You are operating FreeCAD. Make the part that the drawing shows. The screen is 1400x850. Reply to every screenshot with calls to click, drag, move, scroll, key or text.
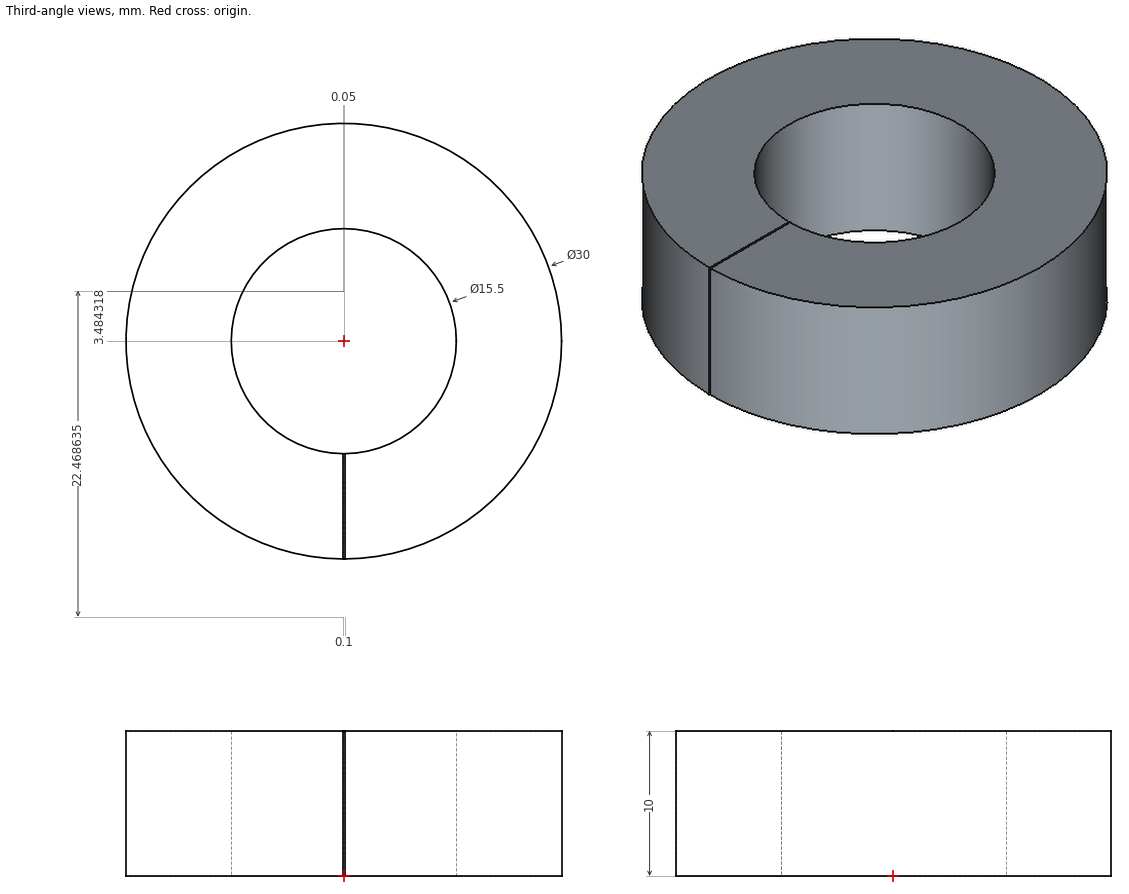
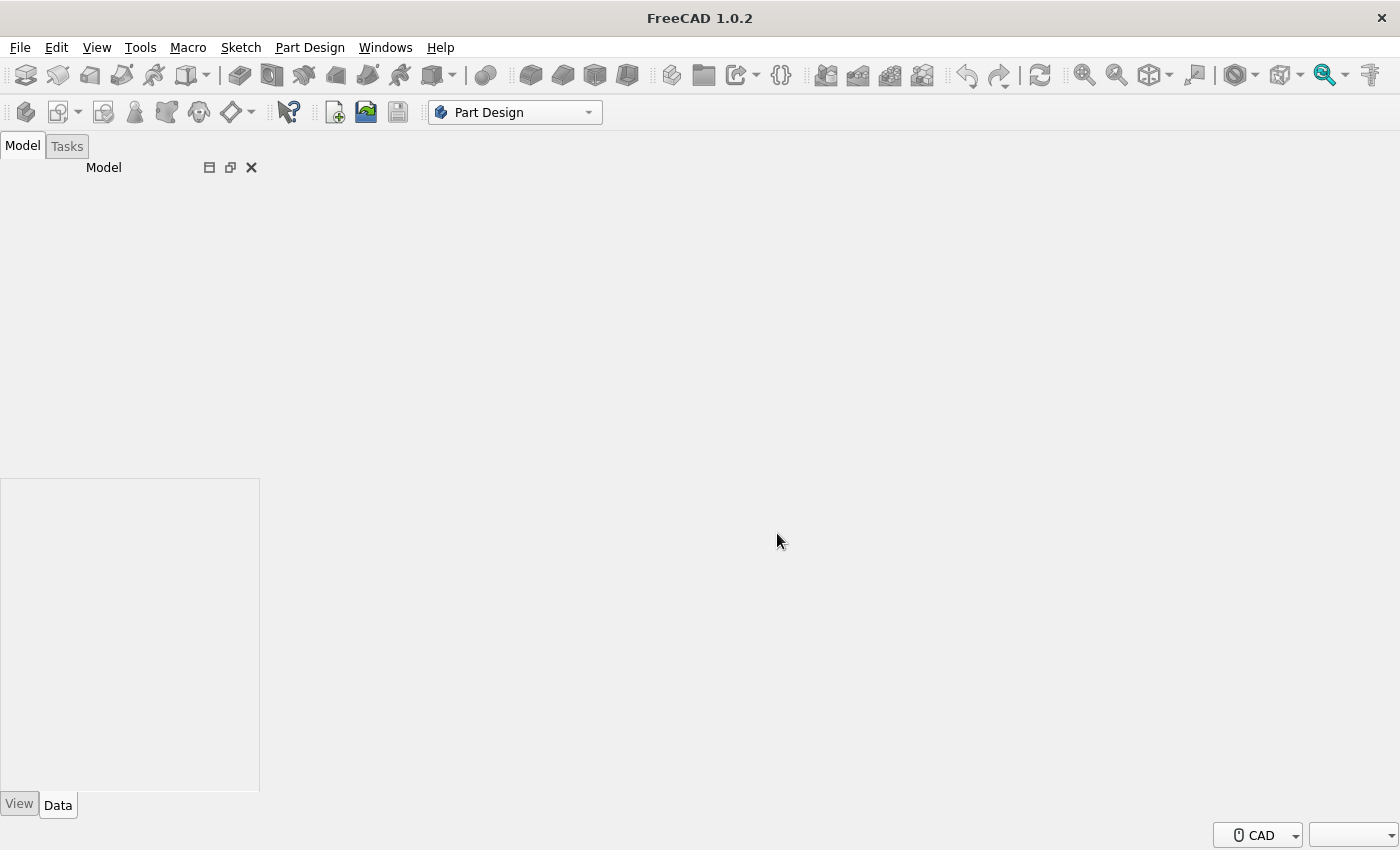
click(334, 112)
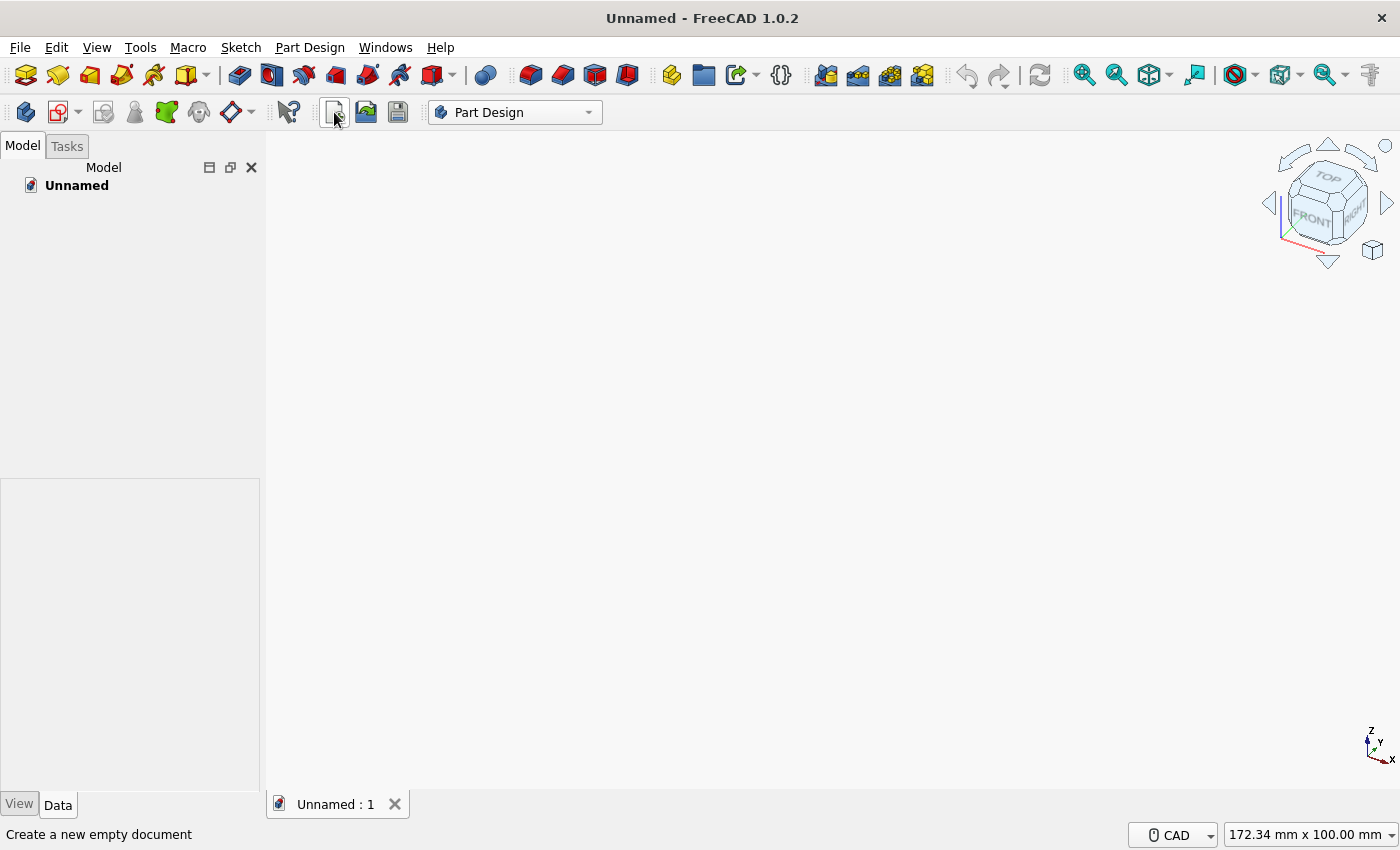
click(58, 112)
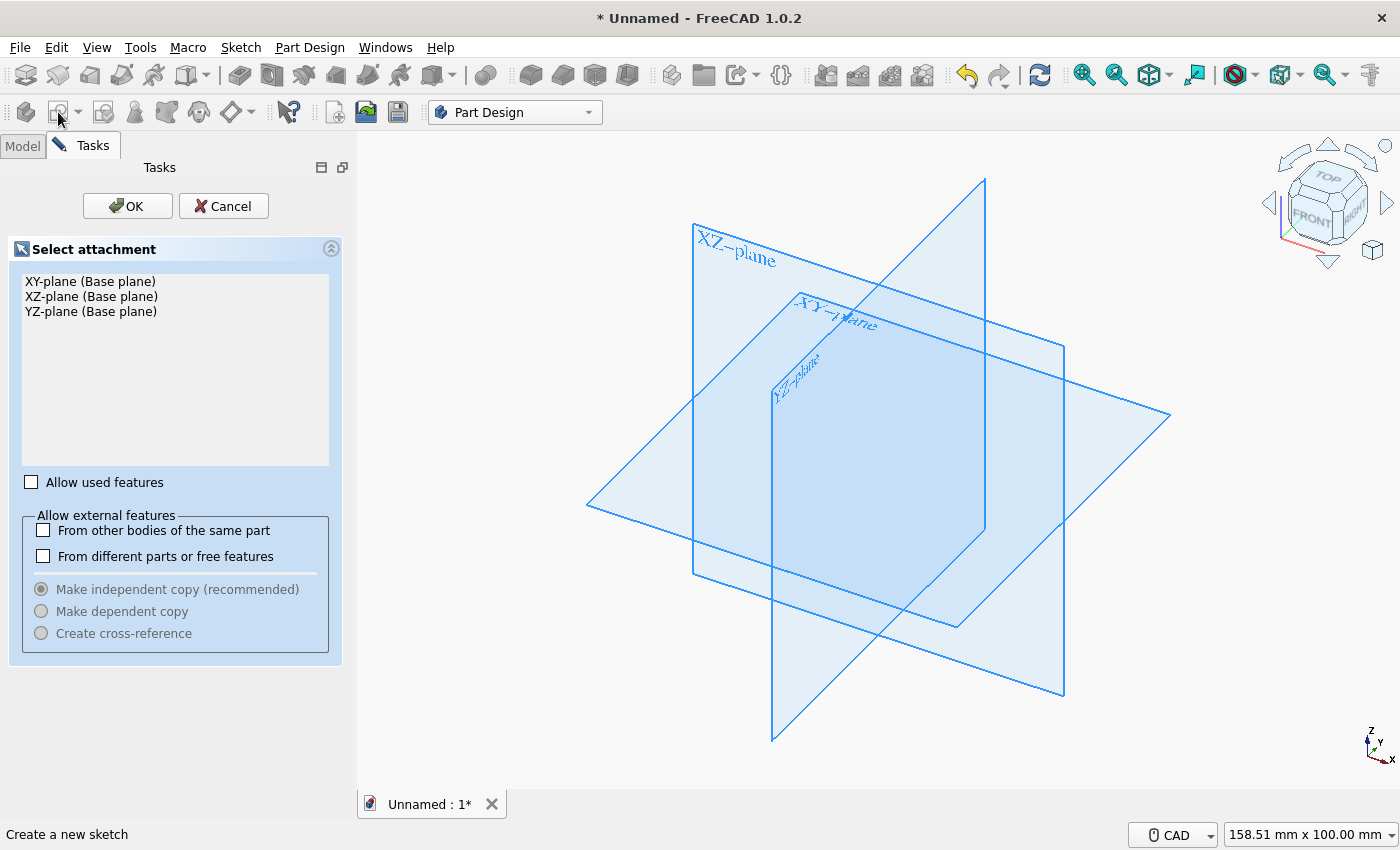
click(82, 282)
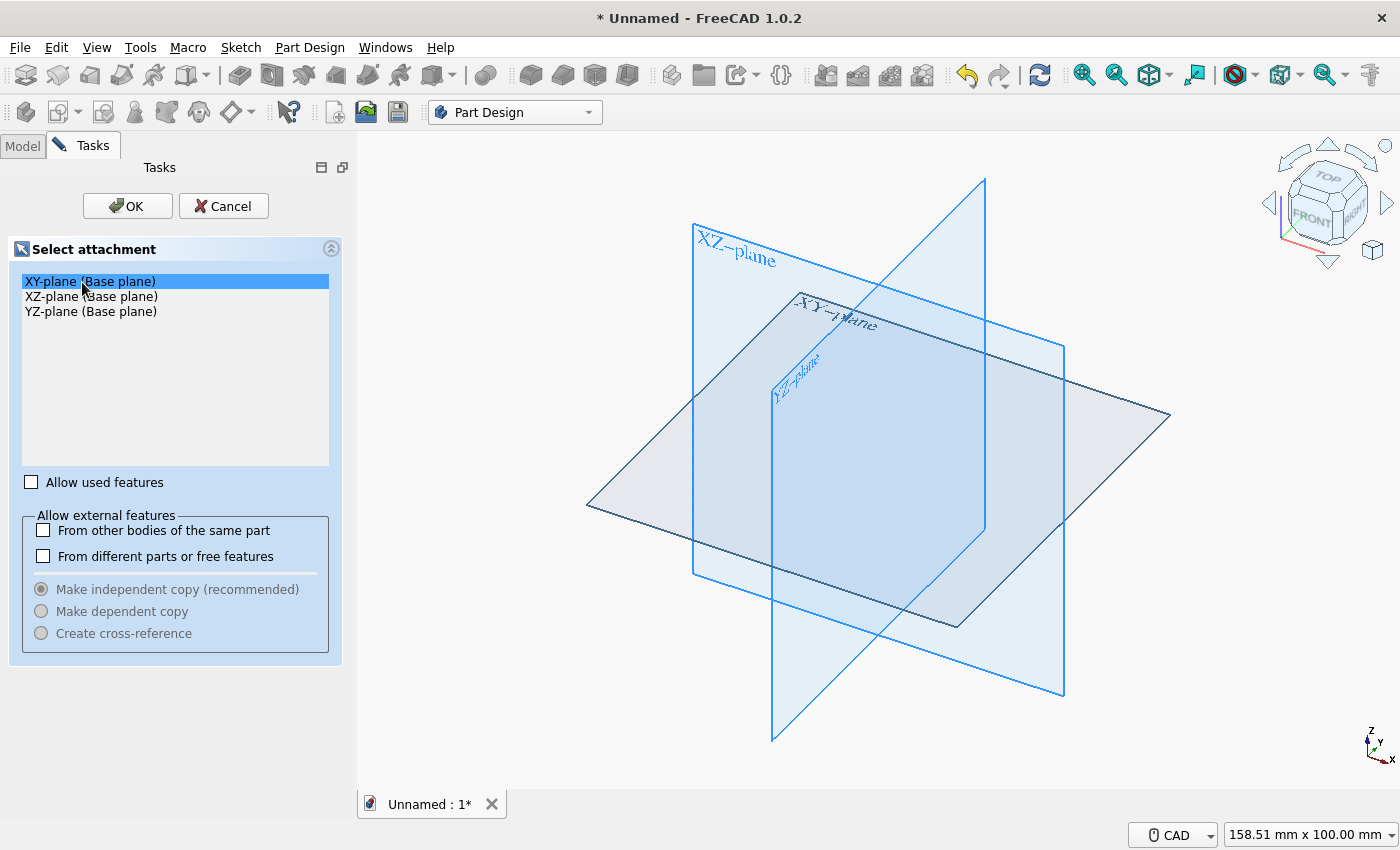
click(128, 206)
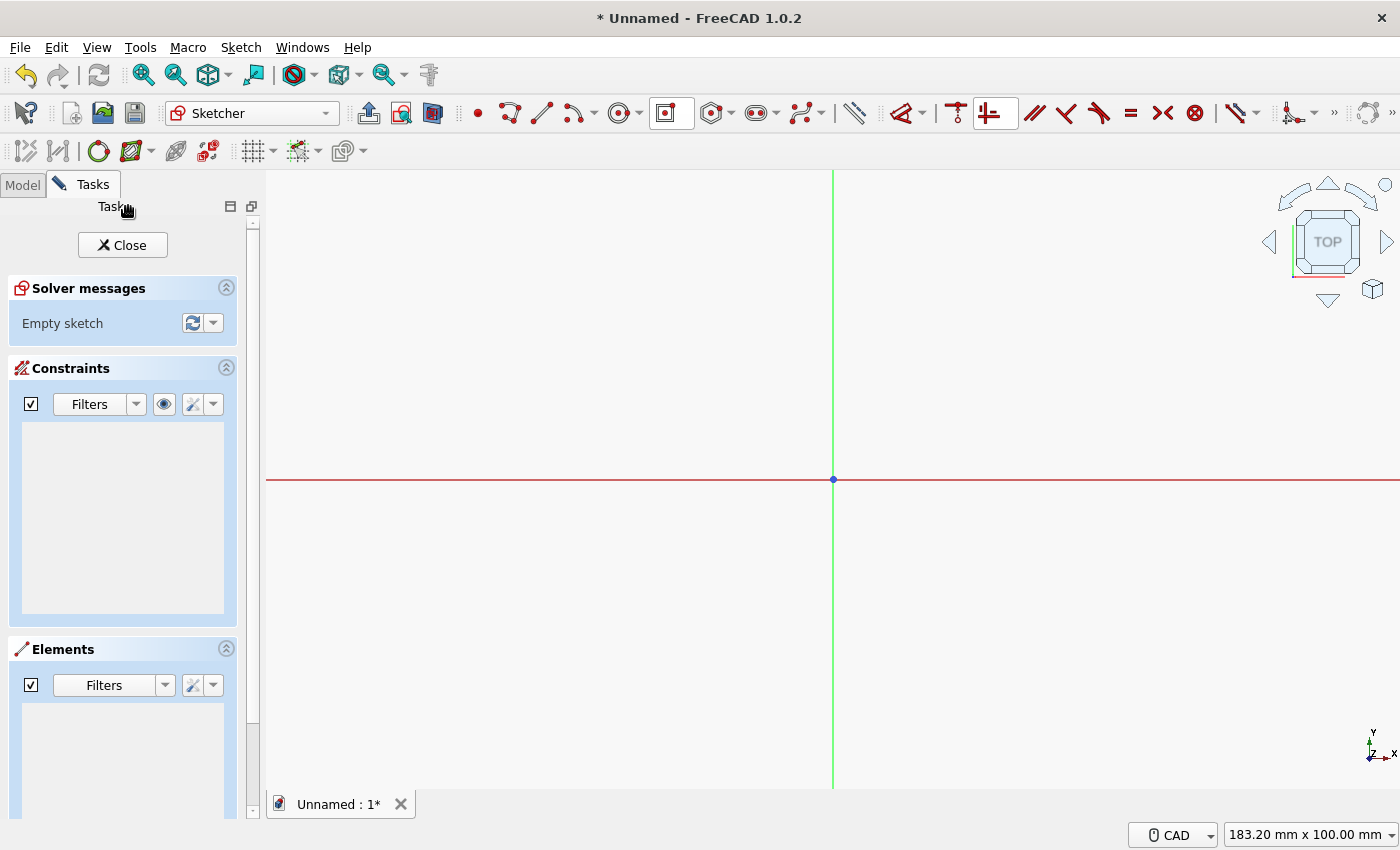
scroll(889, 480, up, 4)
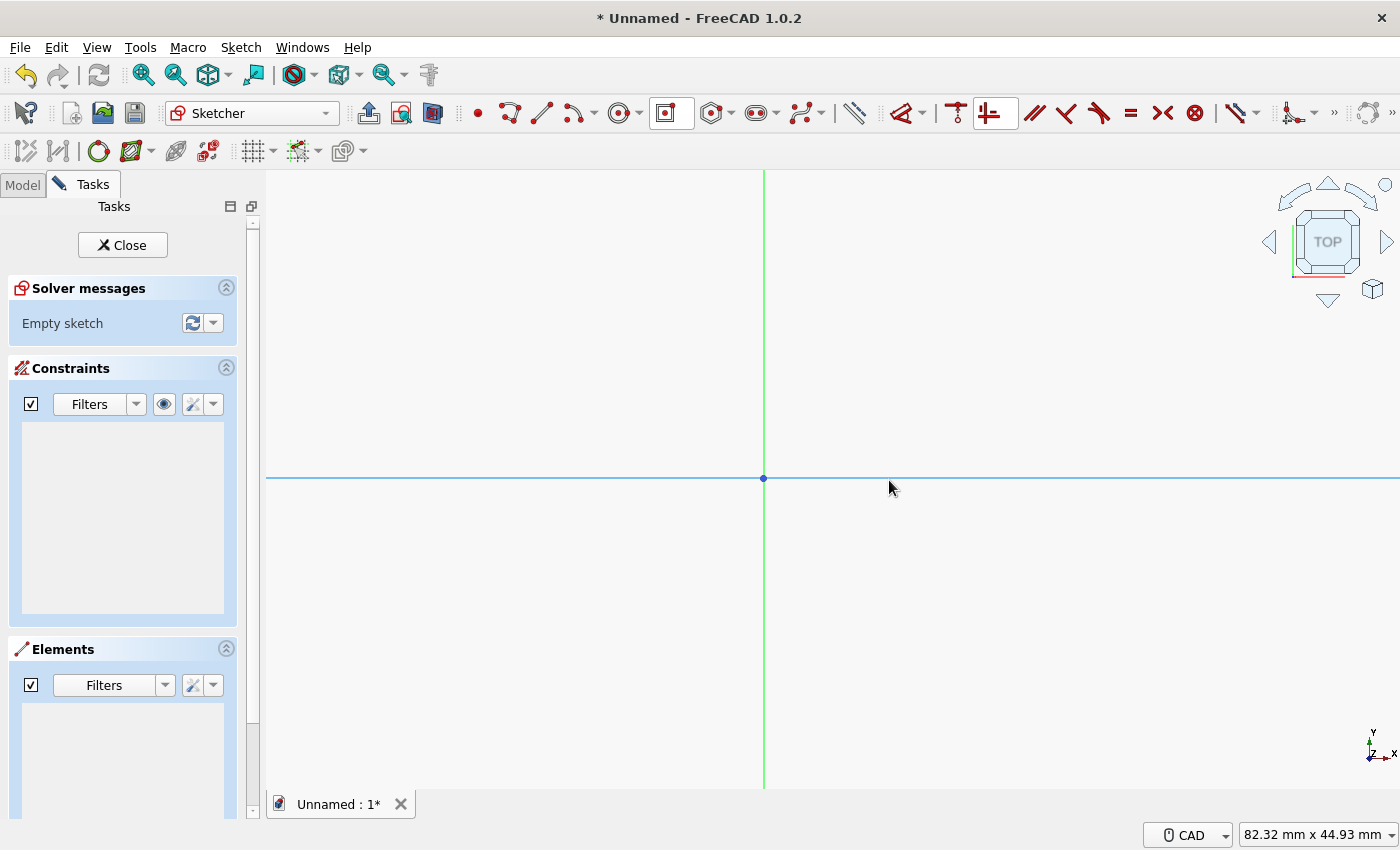
click(620, 114)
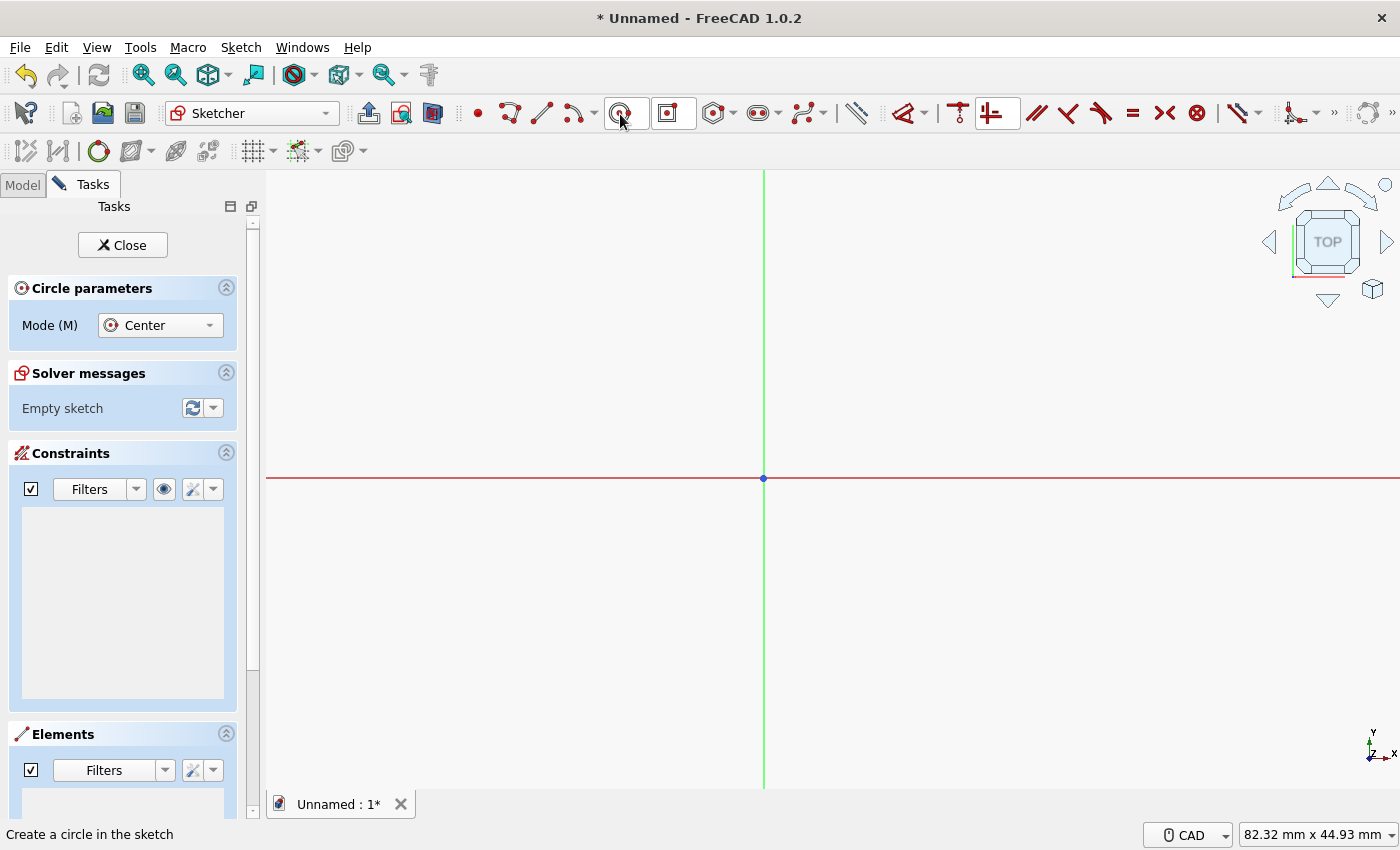
click(764, 478)
move(910, 332)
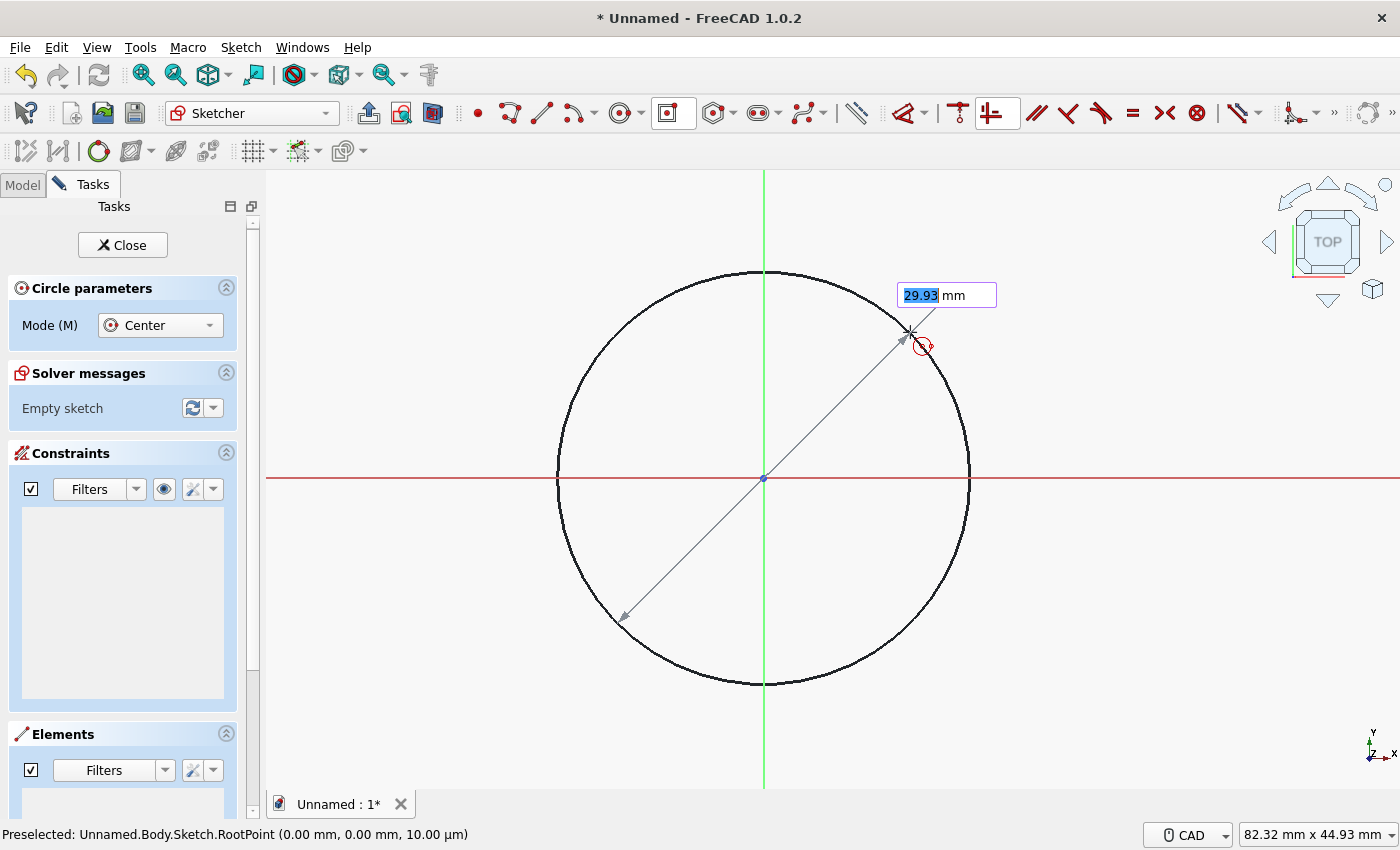
text(30)
key(Return)